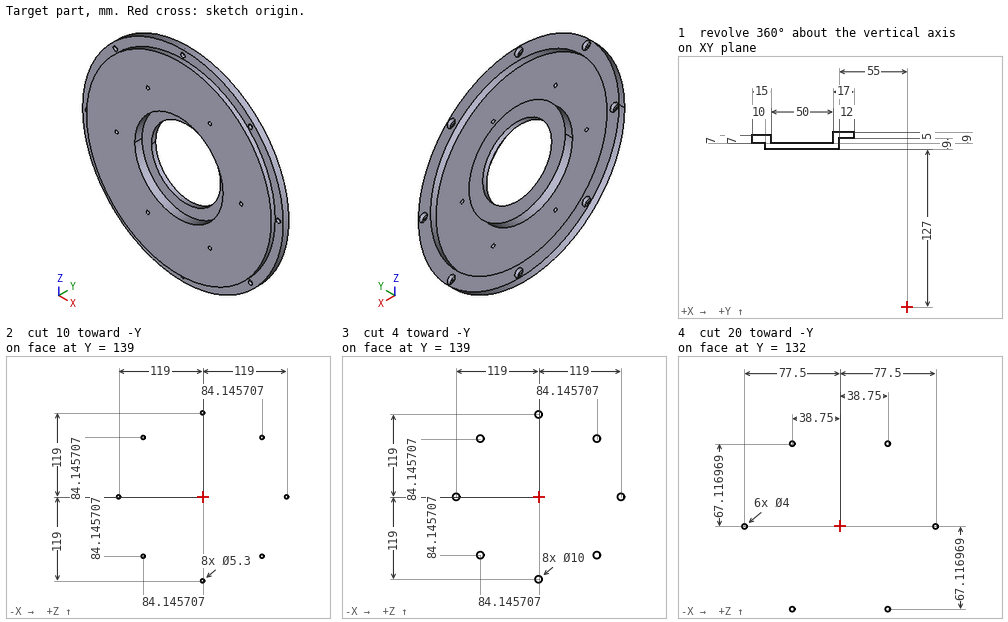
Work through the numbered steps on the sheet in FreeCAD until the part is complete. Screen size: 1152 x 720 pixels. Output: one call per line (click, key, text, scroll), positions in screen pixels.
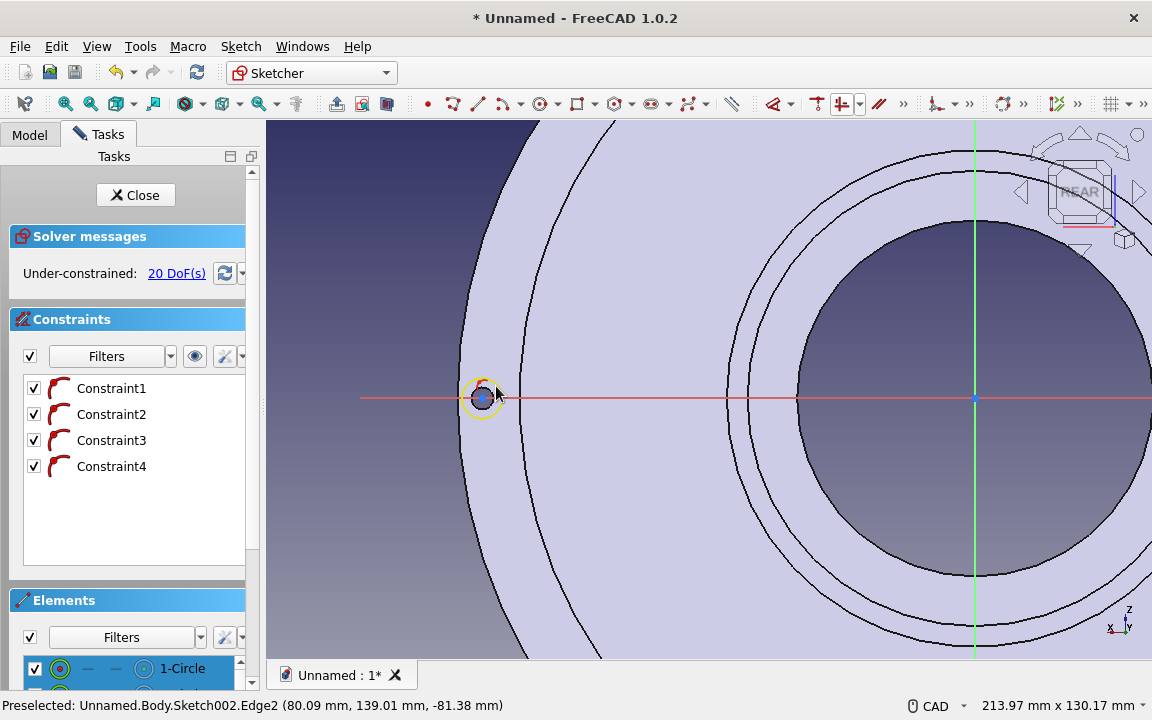
click(496, 384)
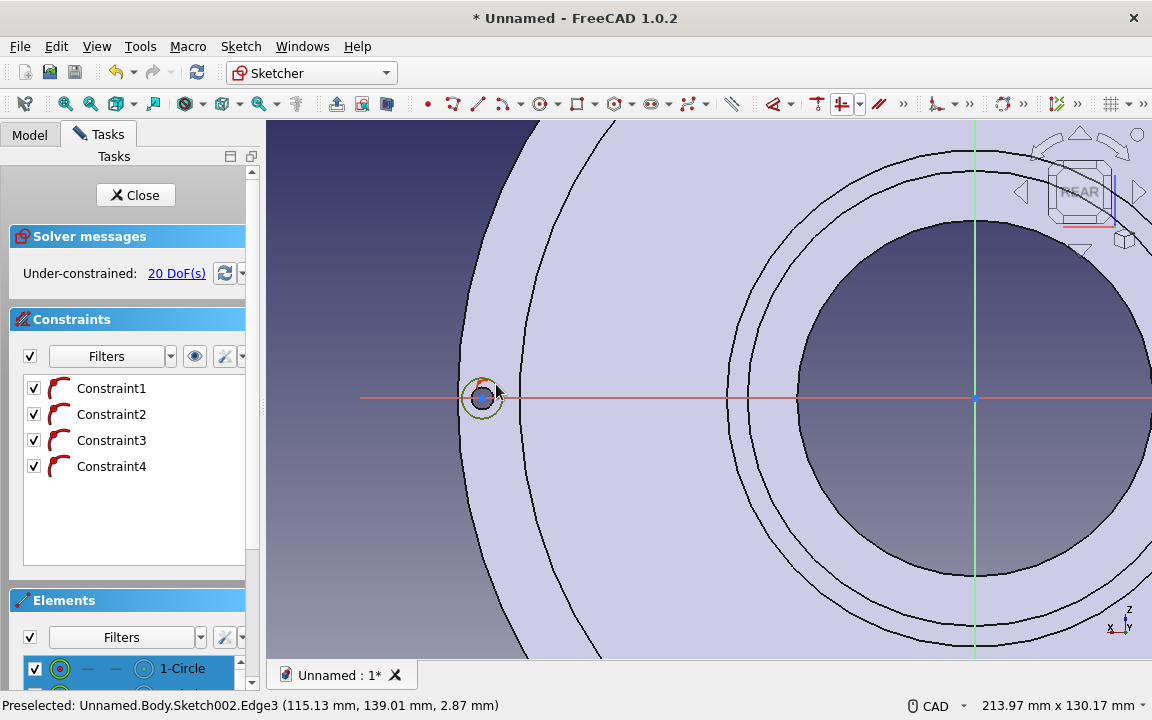
scroll(496, 386, down, 6)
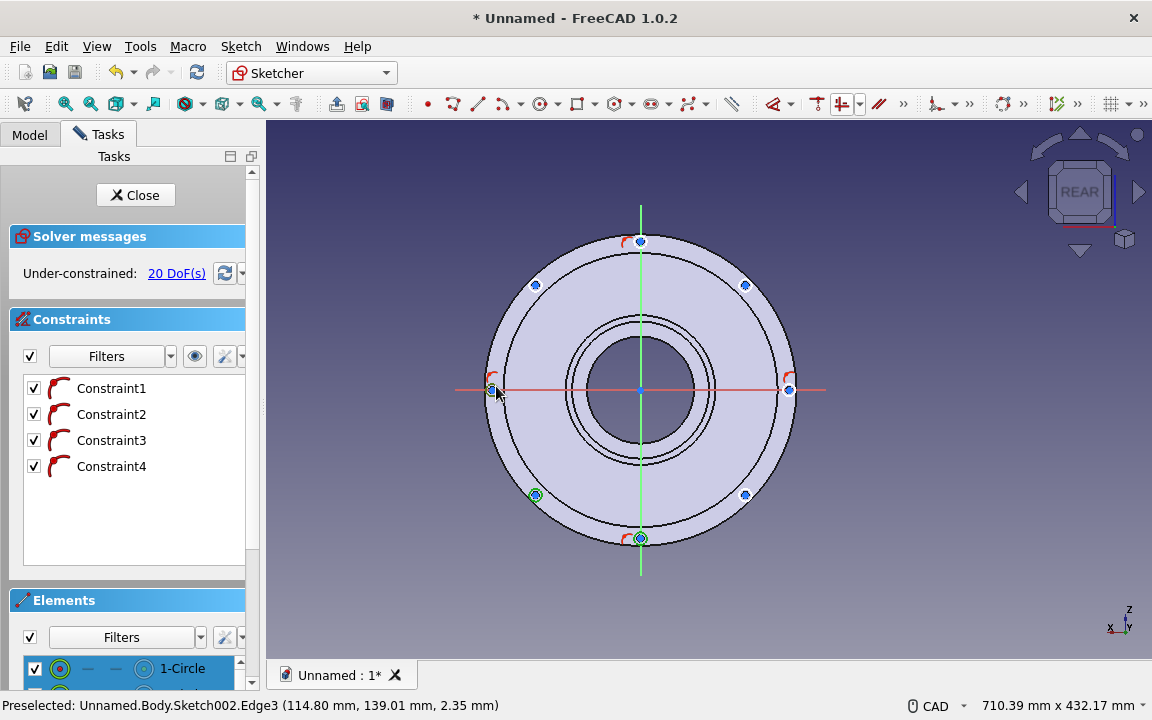
scroll(540, 281, up, 4)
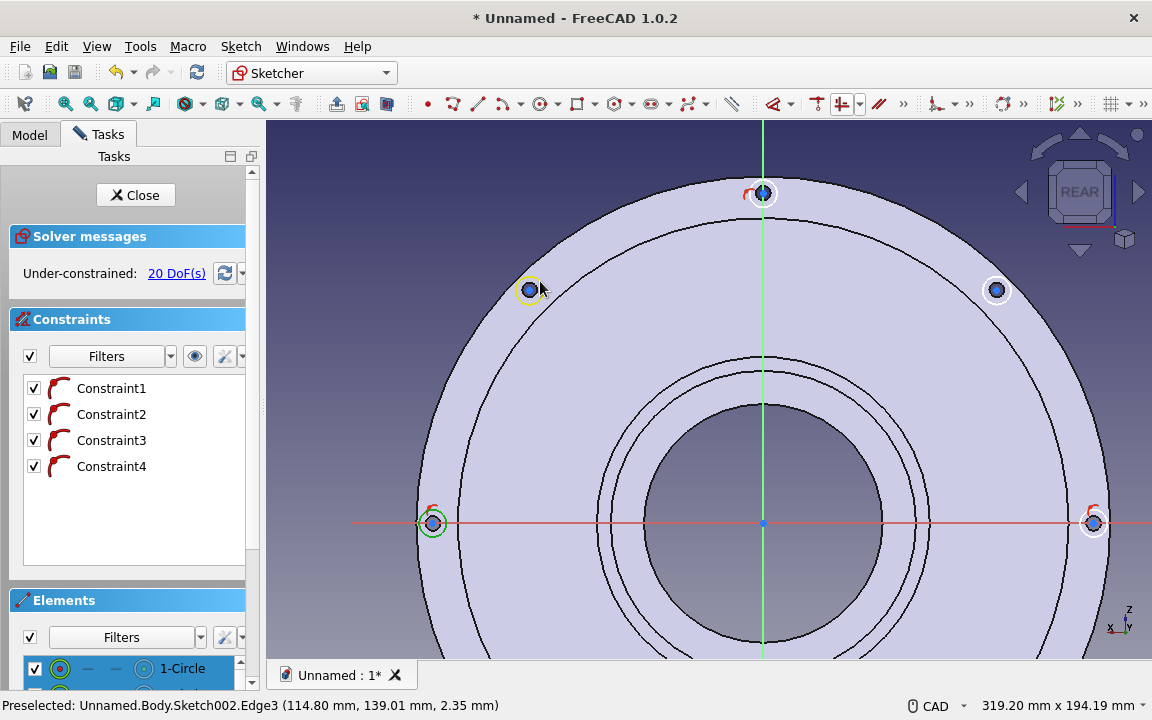
click(540, 281)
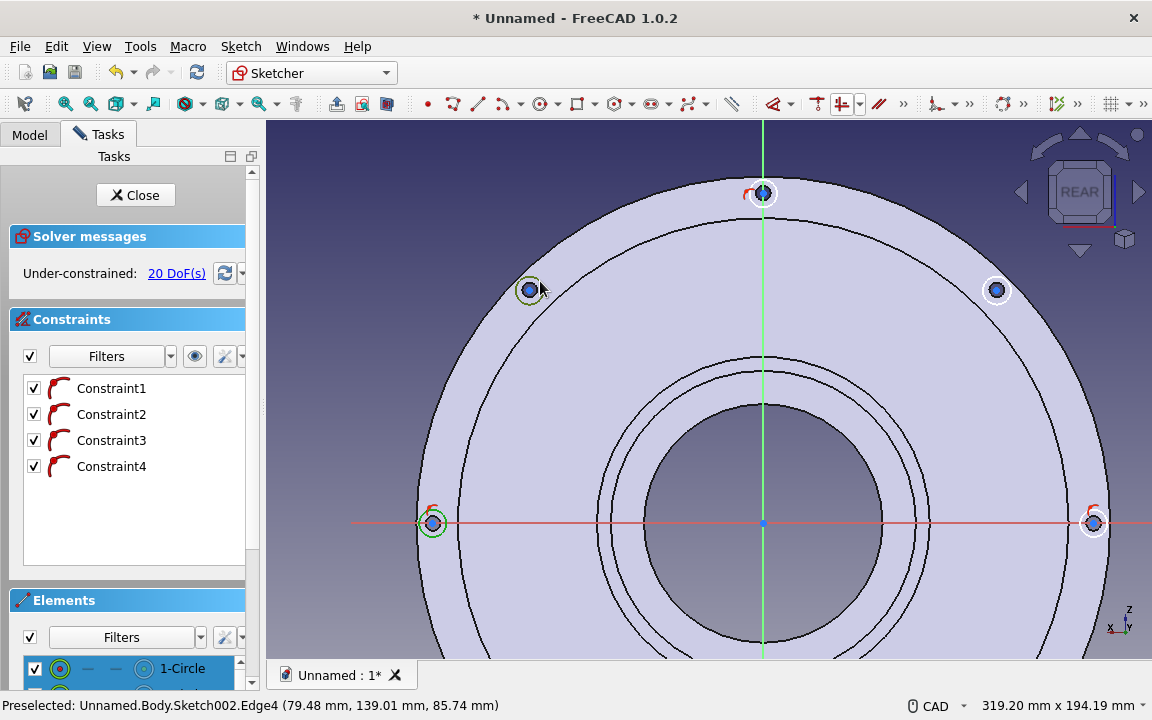
scroll(773, 184, up, 2)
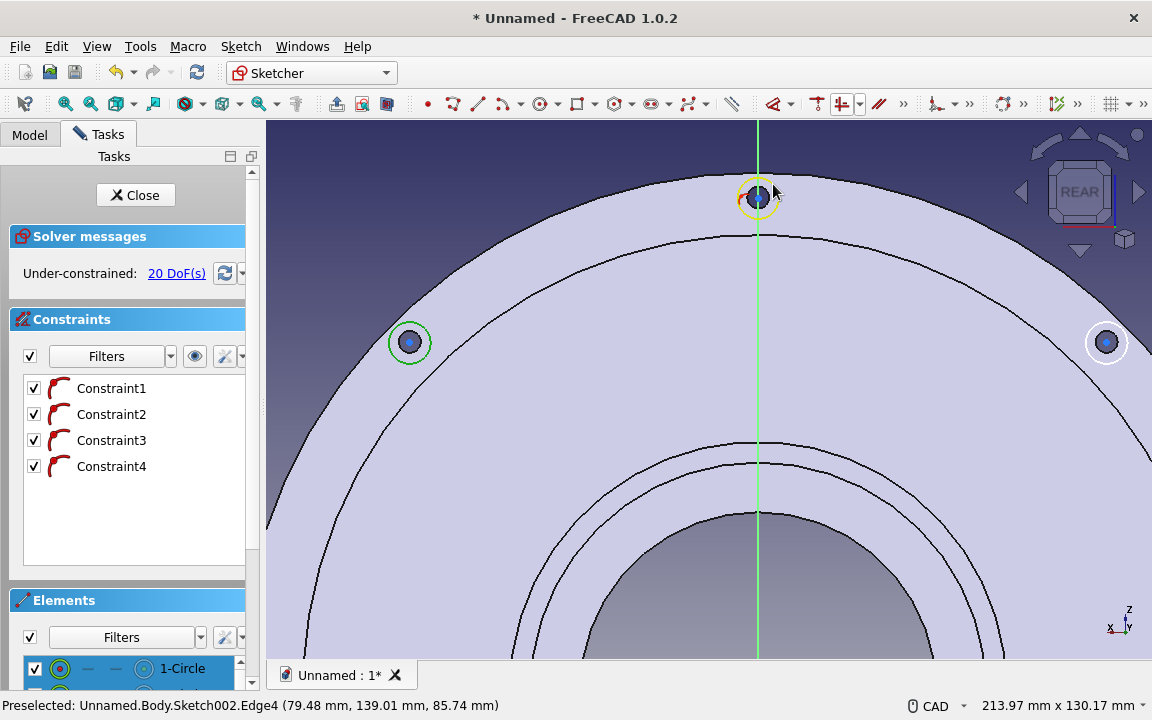
click(773, 184)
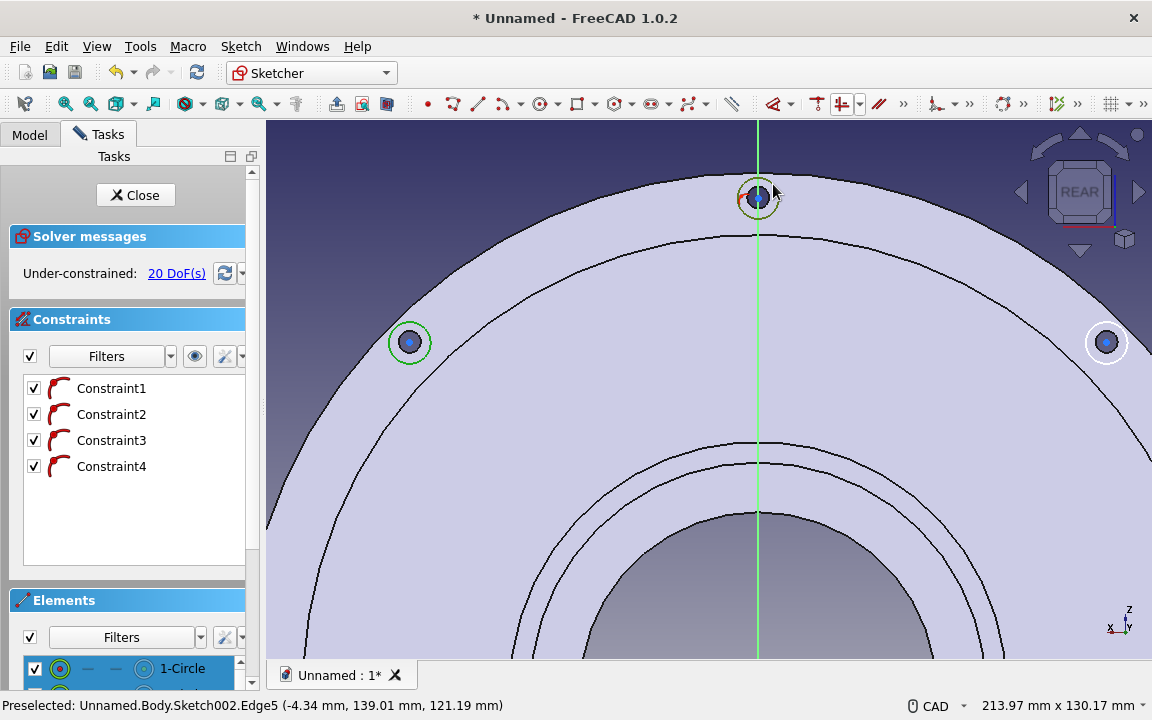
scroll(590, 260, down, 6)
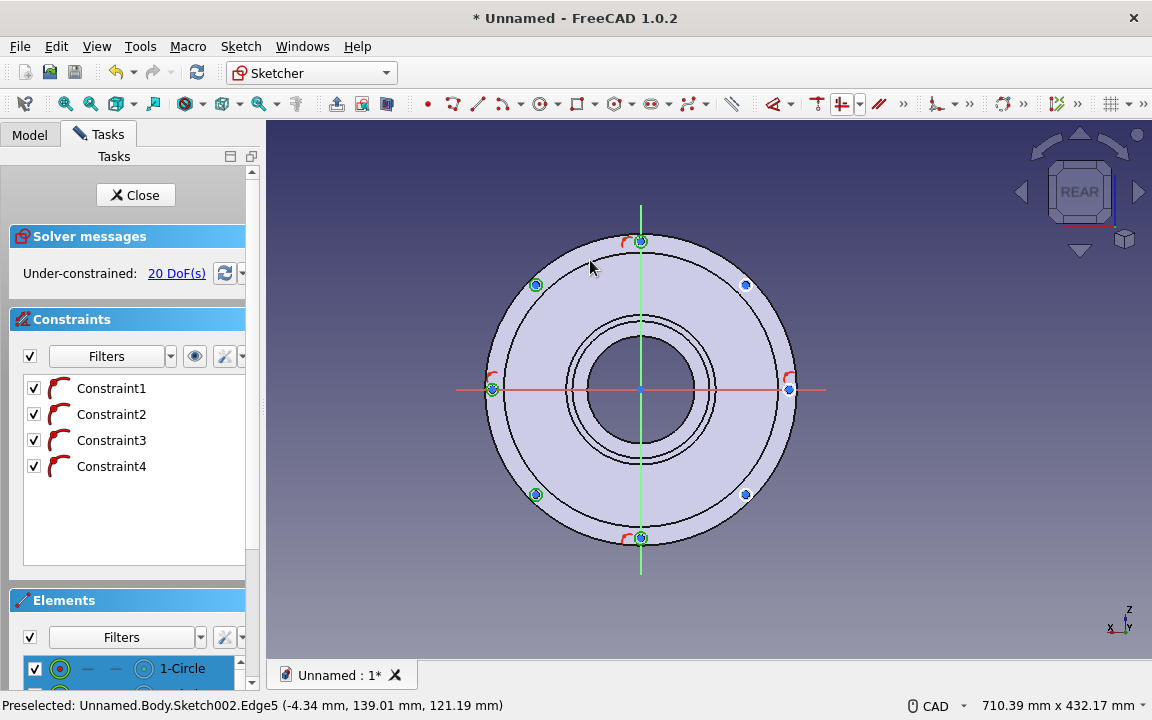
scroll(750, 281, up, 4)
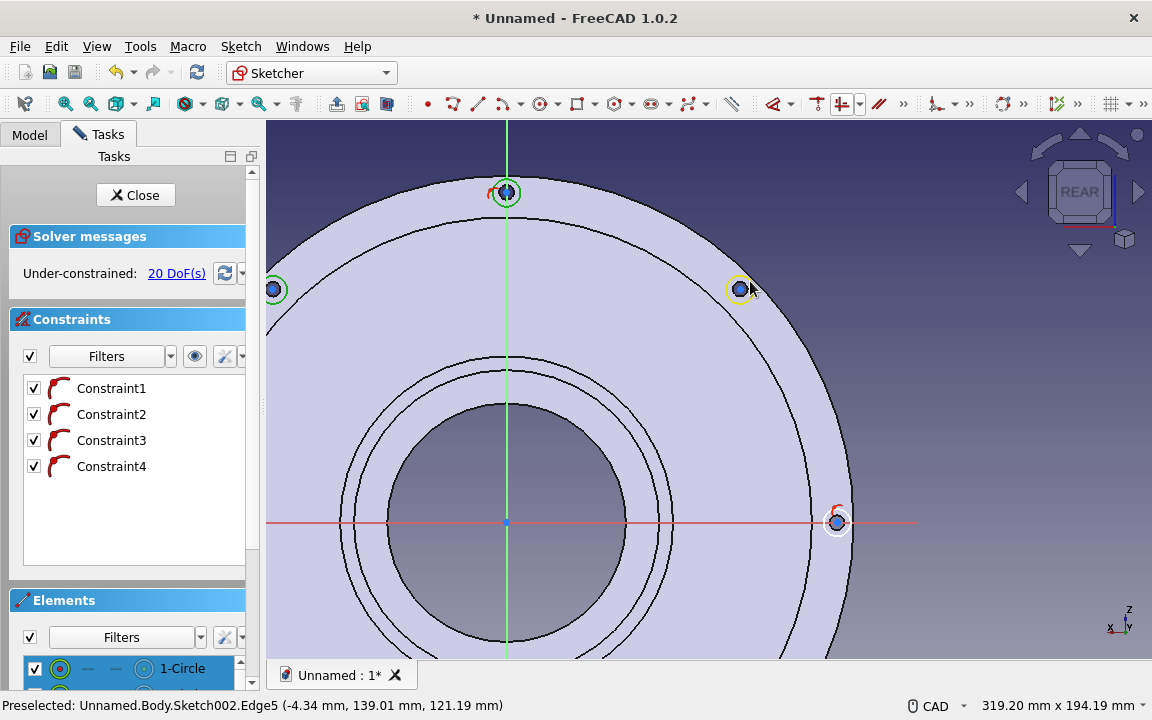
click(750, 280)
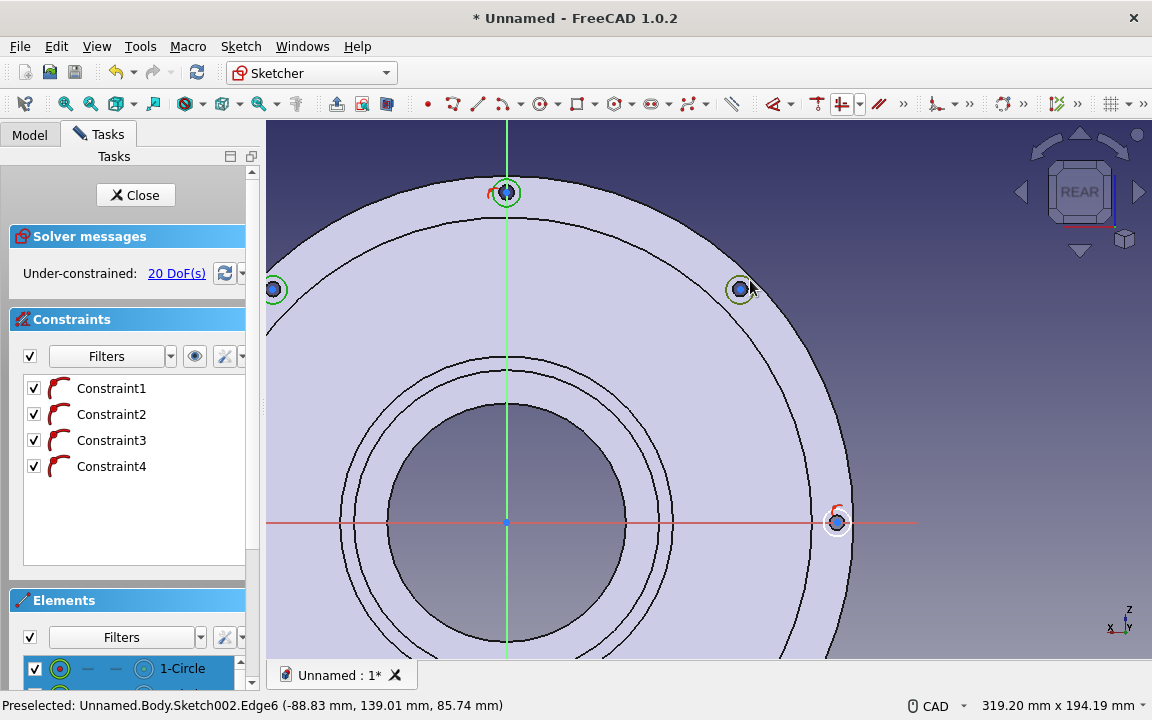
scroll(847, 513, up, 2)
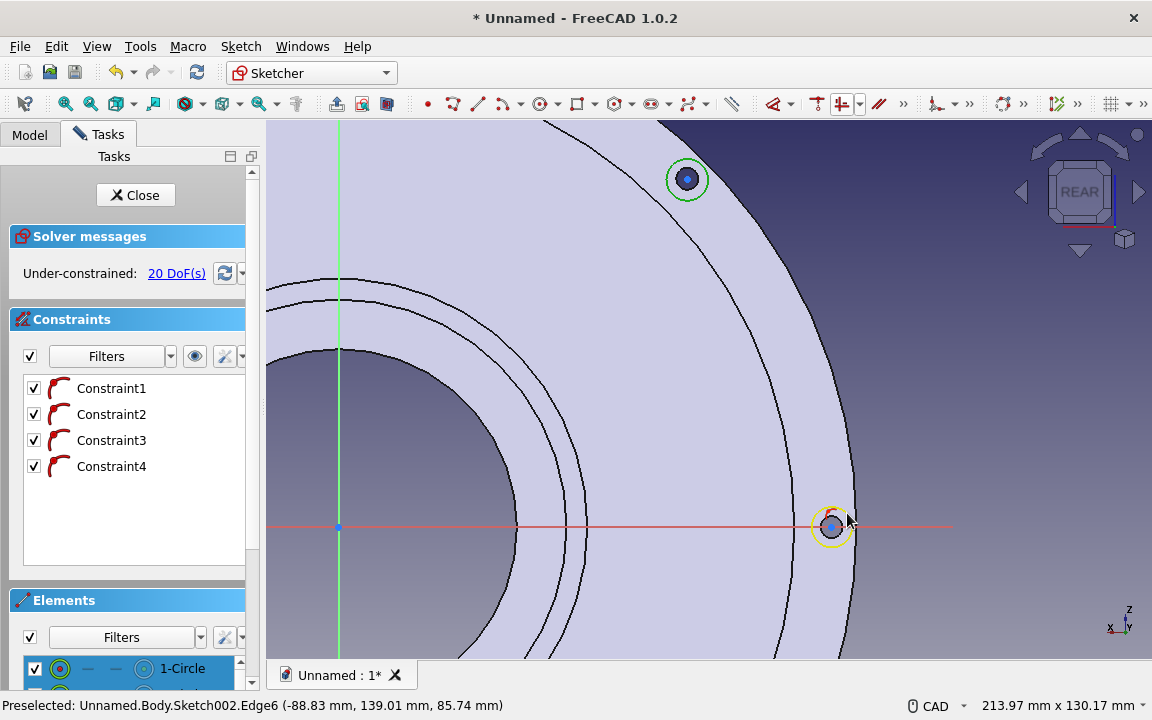
click(846, 513)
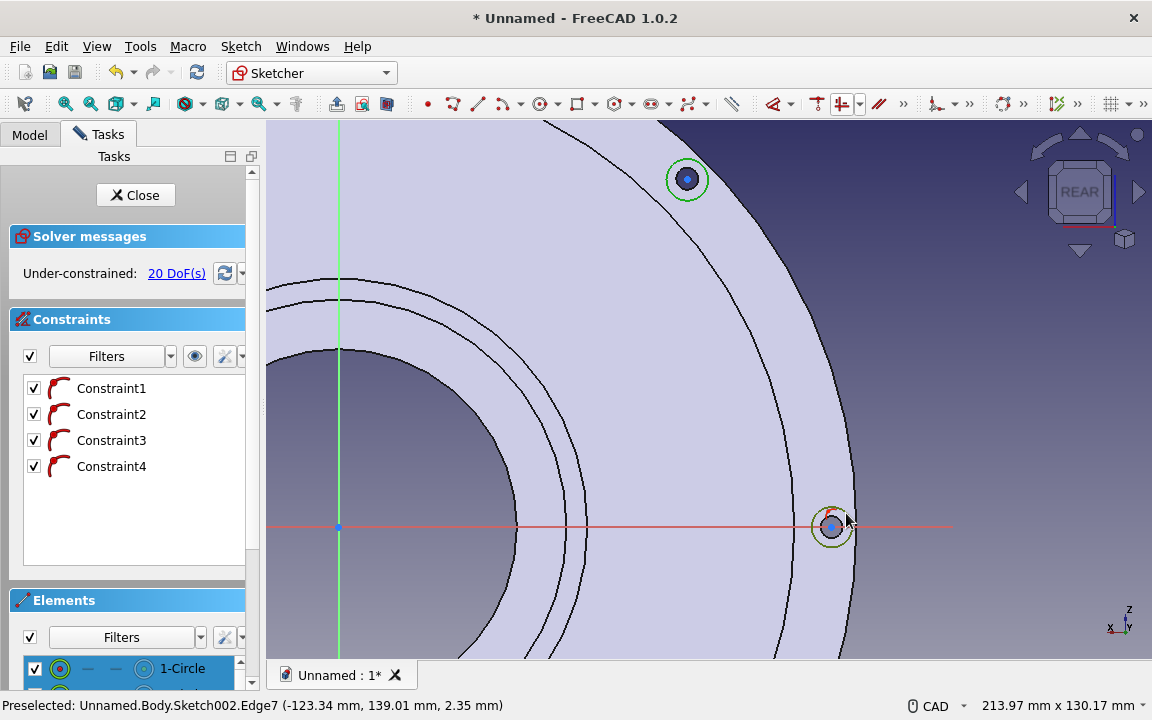
scroll(771, 330, down, 6)